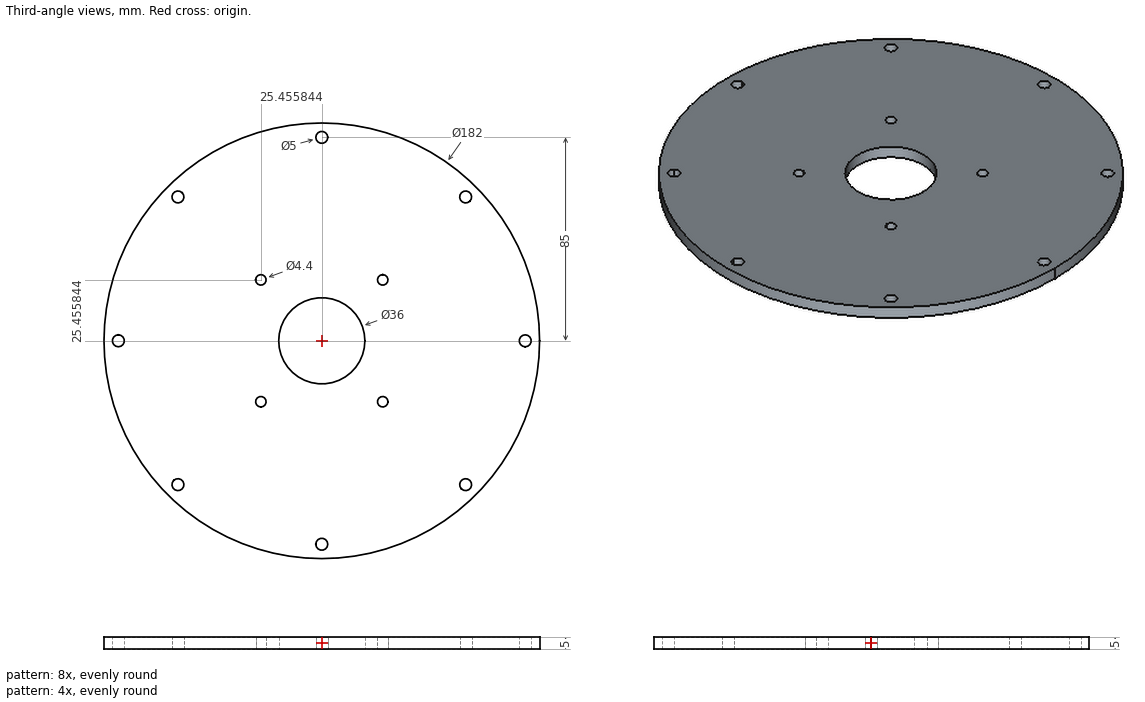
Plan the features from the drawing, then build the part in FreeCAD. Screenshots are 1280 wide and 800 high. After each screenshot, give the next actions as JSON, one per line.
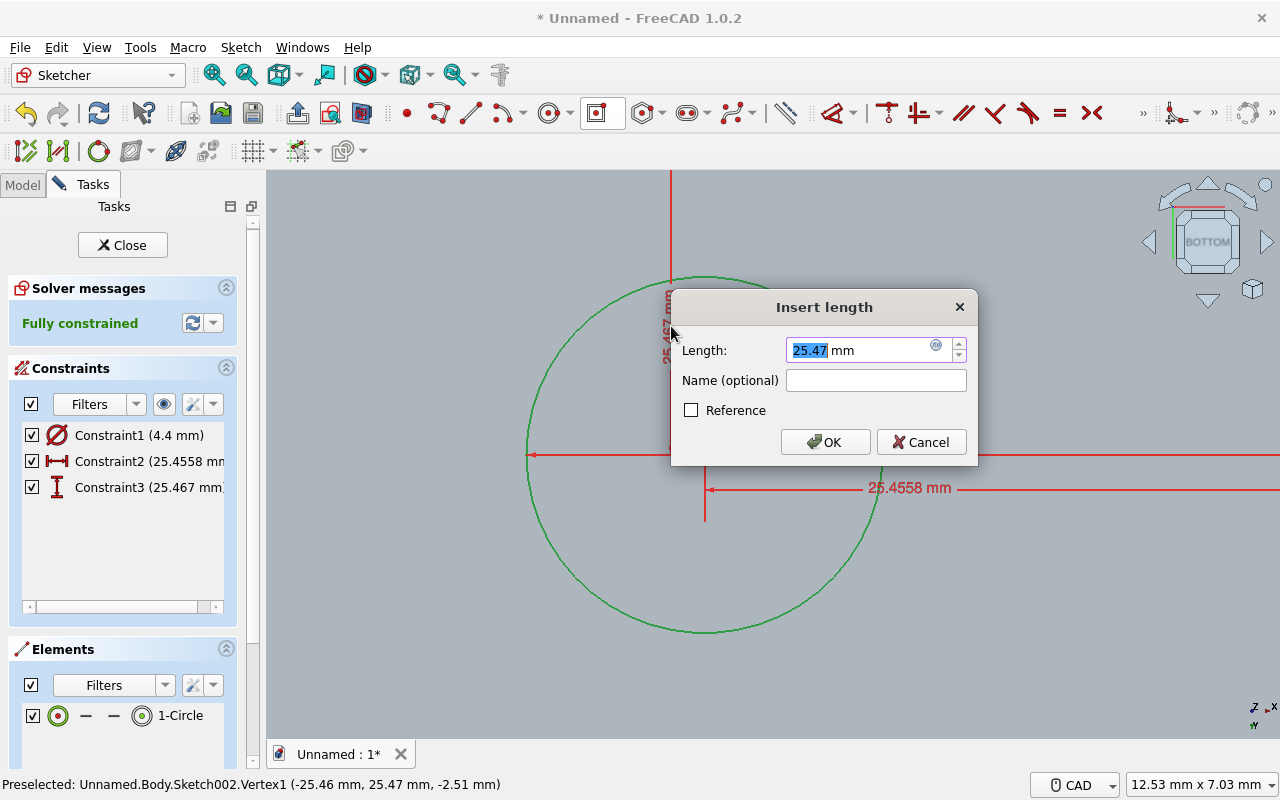
{"action": "type", "text": "25.455844"}
{"action": "key", "text": "Return"}
{"action": "key", "text": "Escape"}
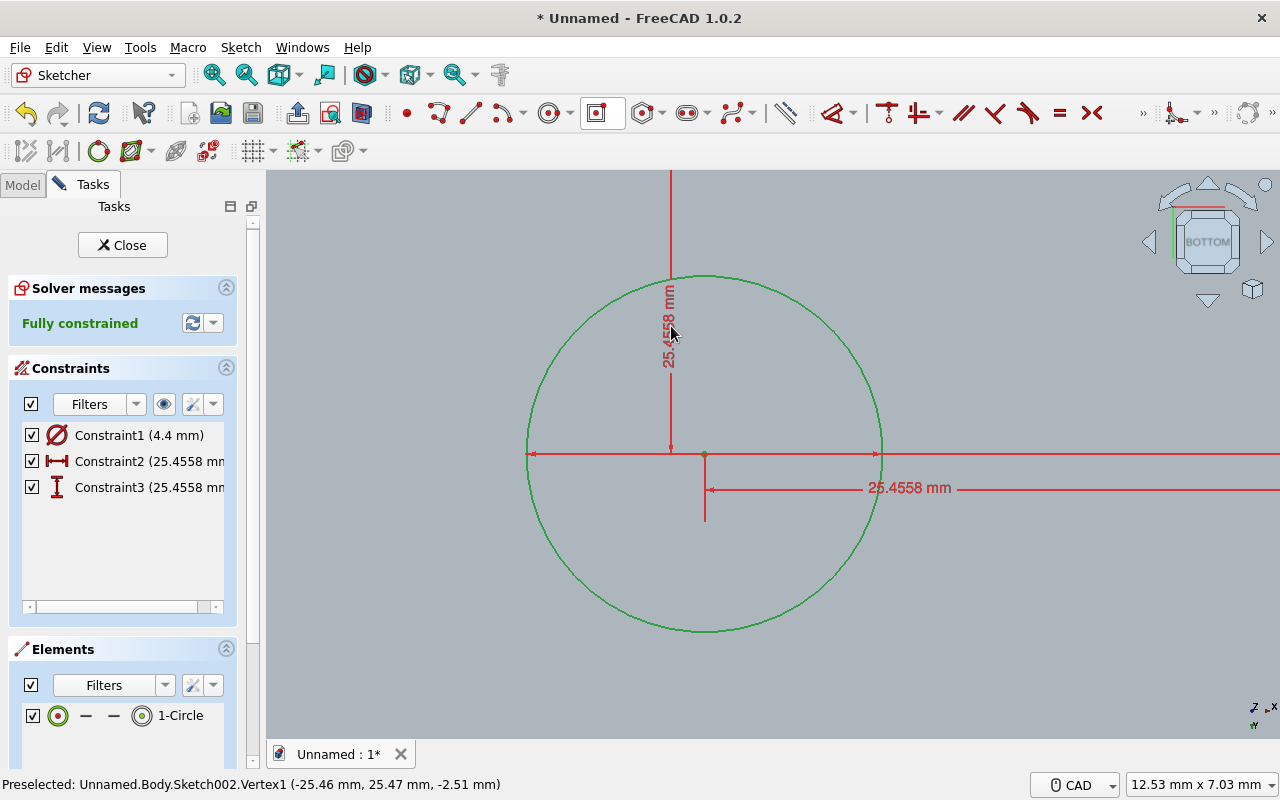
{"action": "left_click", "coordinate": [123, 245]}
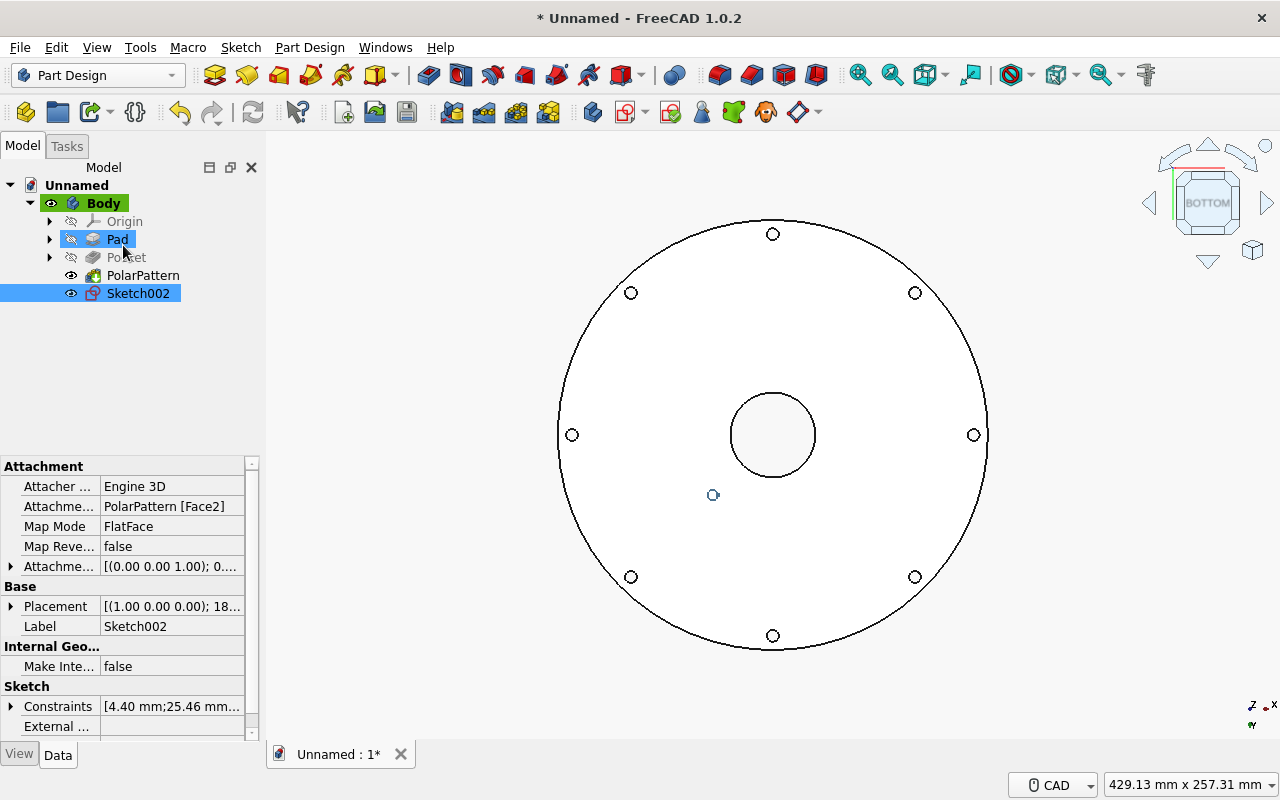
{"action": "left_click", "coordinate": [430, 76]}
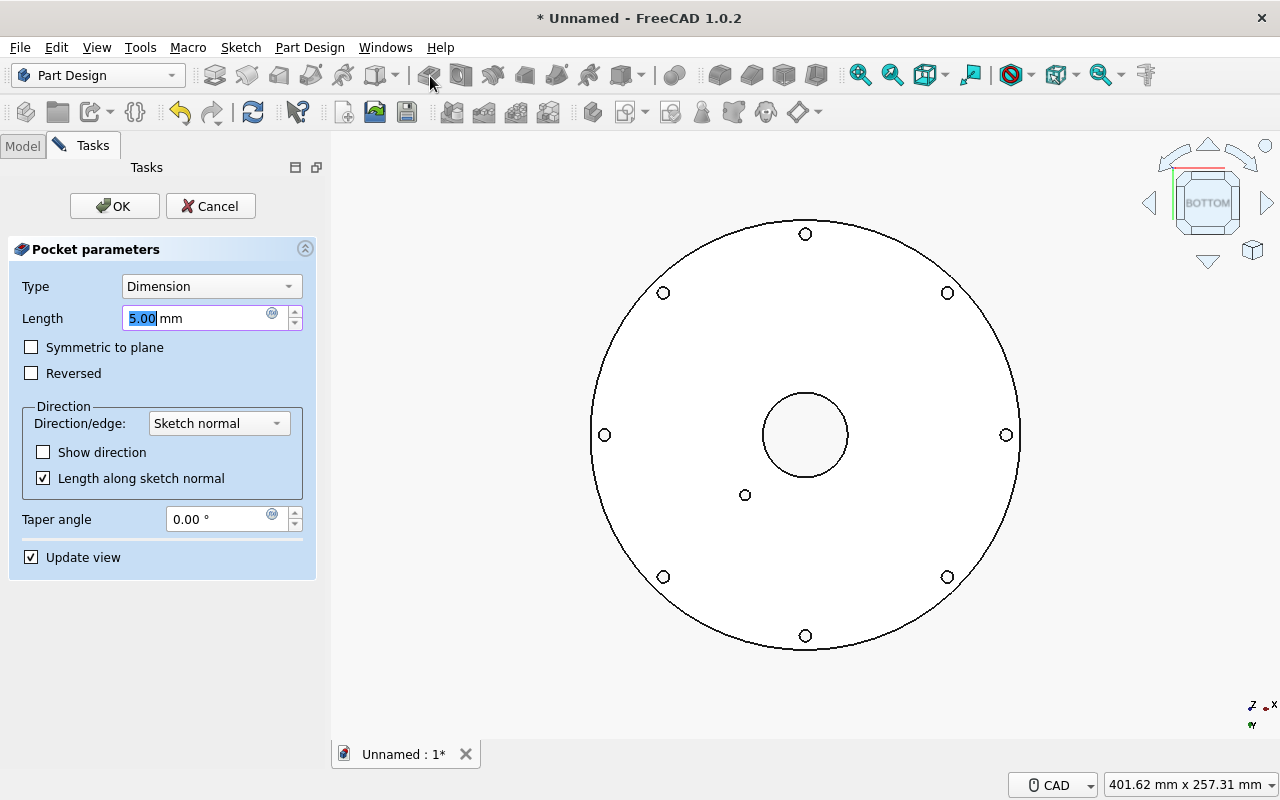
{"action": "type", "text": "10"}
{"action": "key", "text": "Tab"}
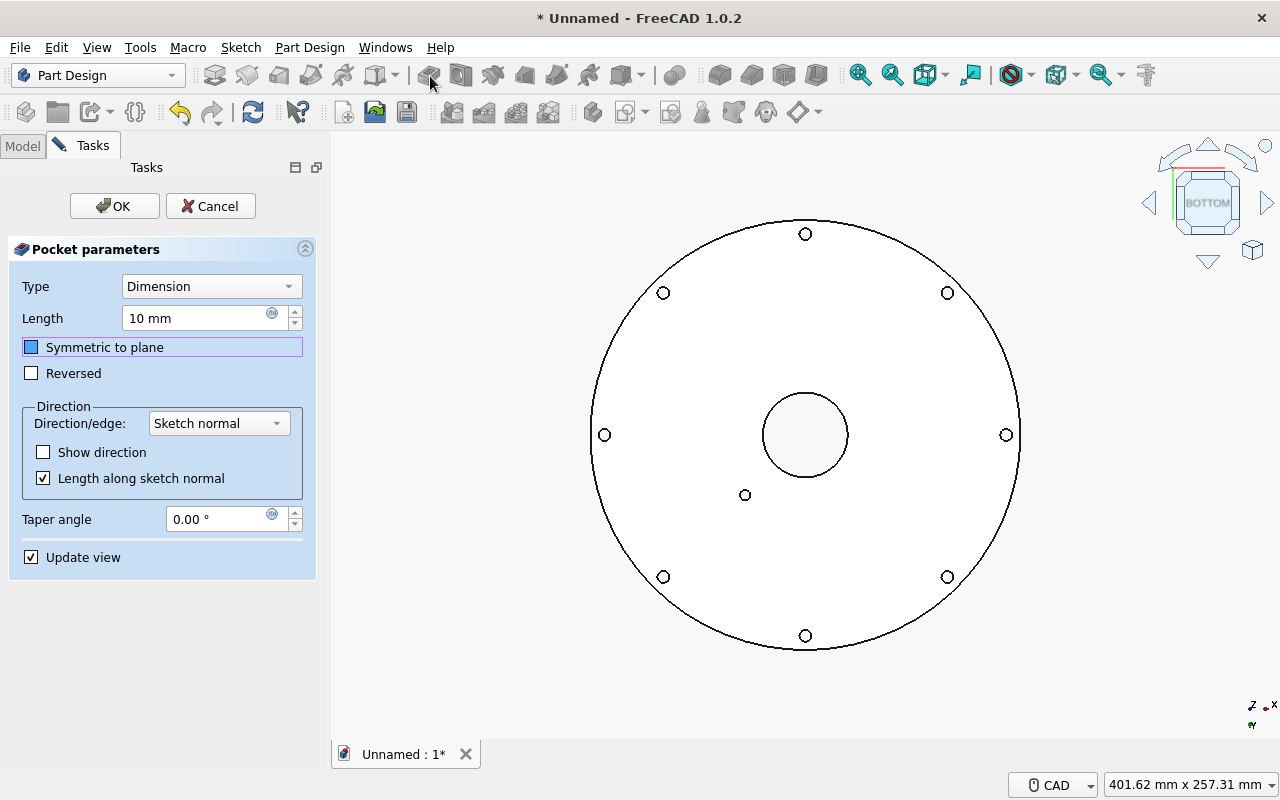
{"action": "left_click", "coordinate": [115, 206]}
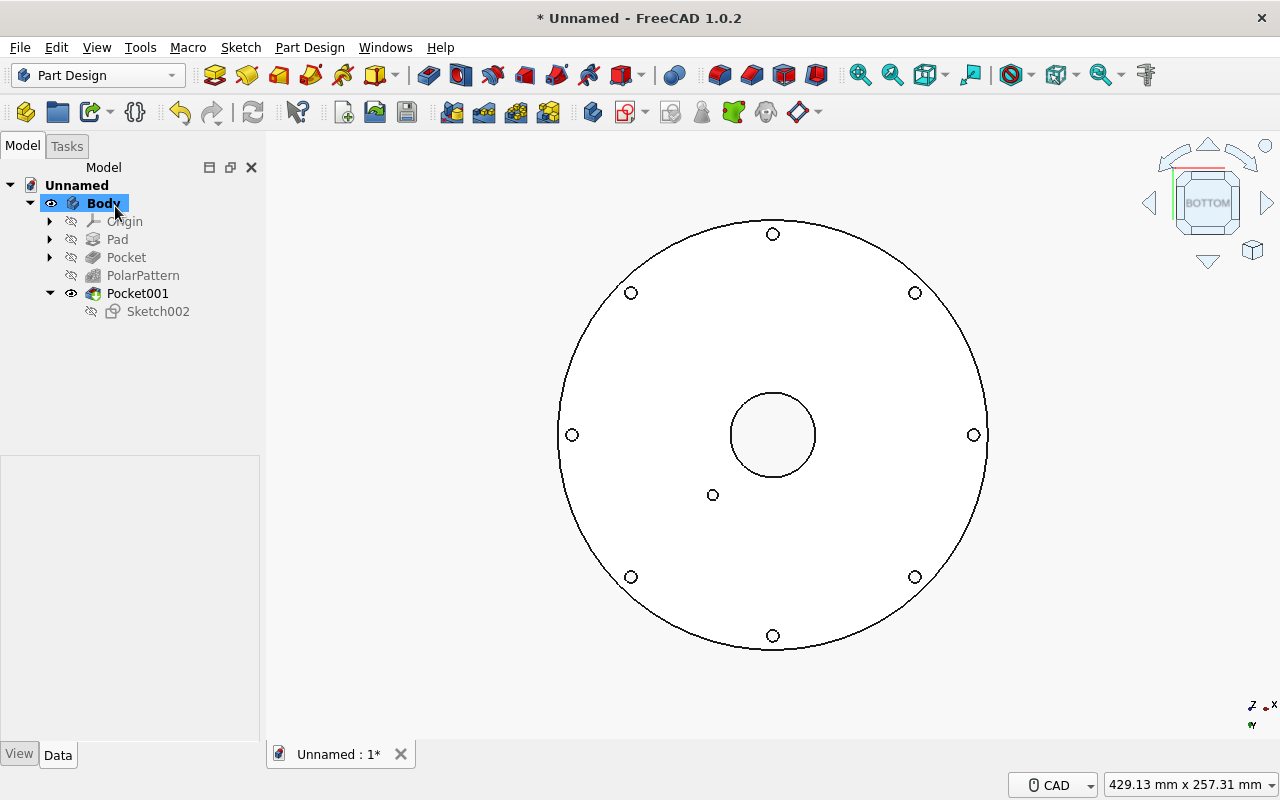
{"action": "left_click", "coordinate": [116, 293]}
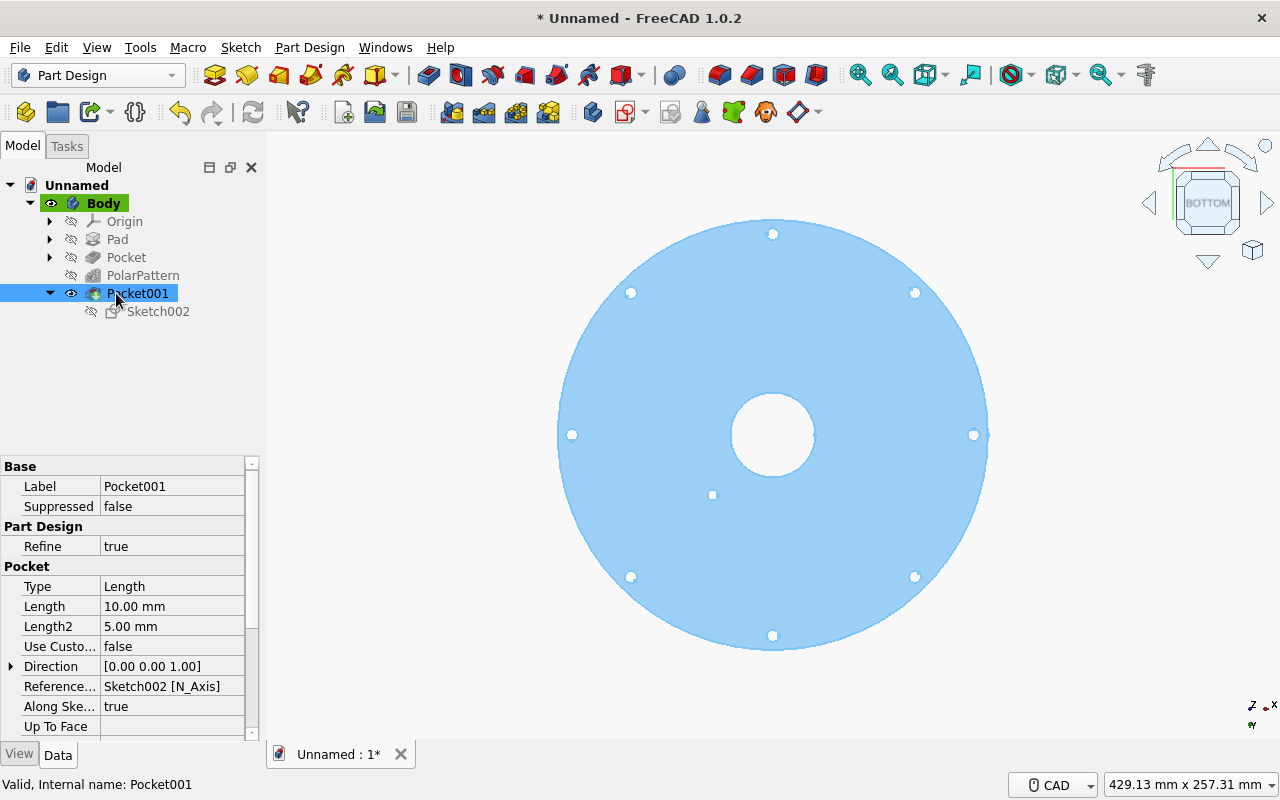
{"action": "left_click", "coordinate": [516, 112]}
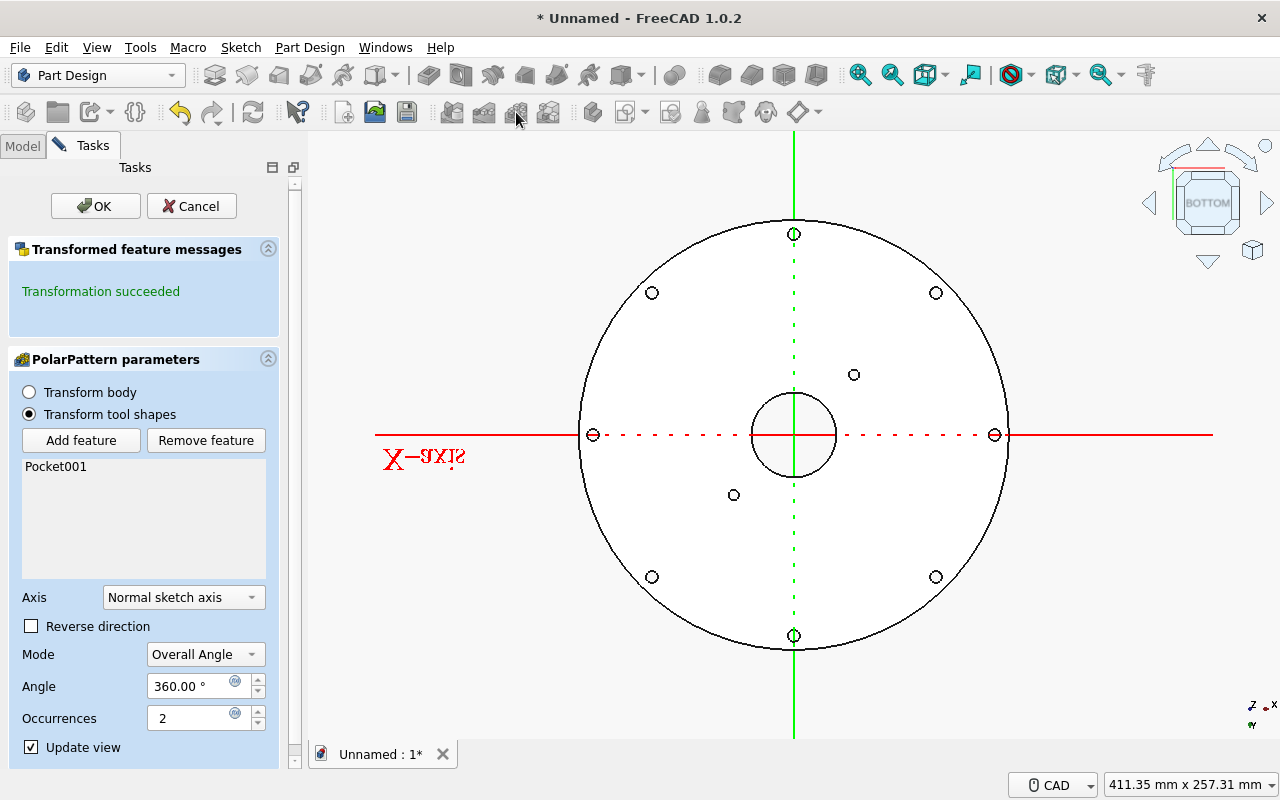
{"action": "left_click", "coordinate": [184, 598]}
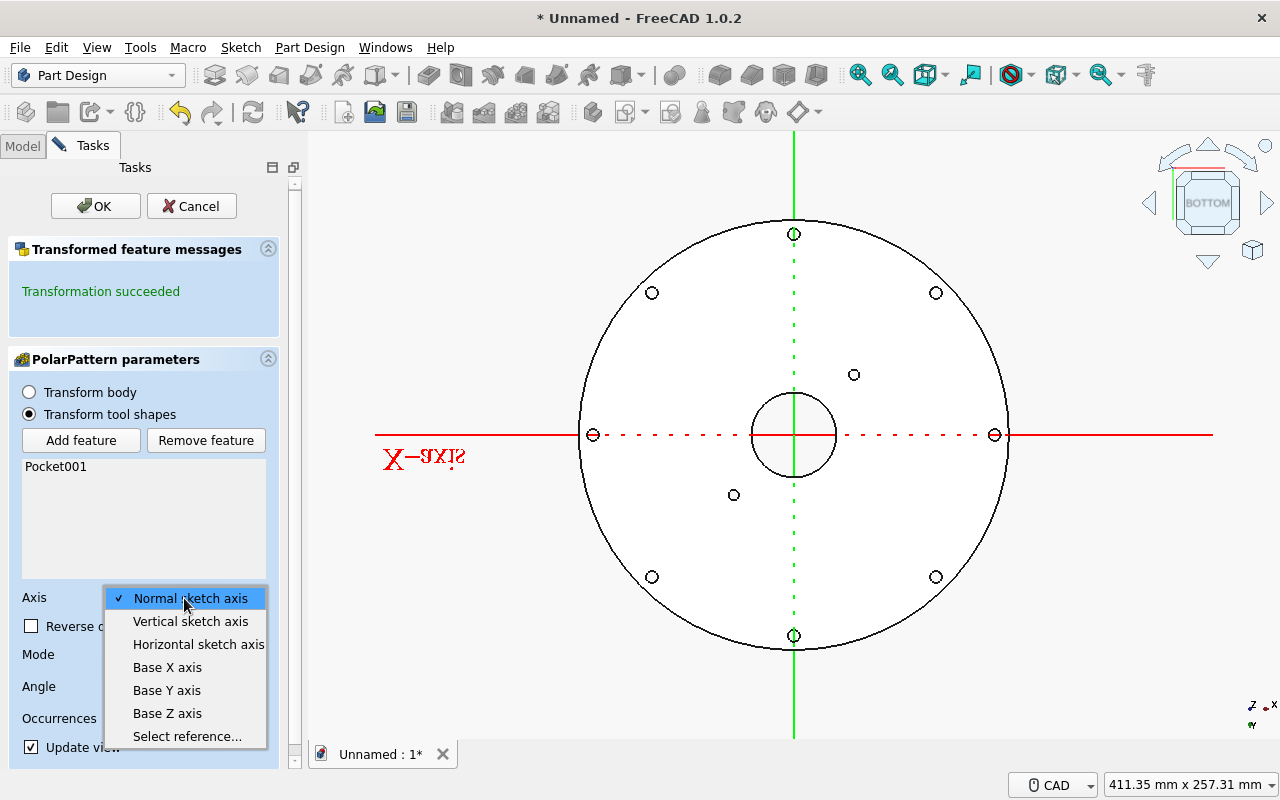
{"action": "left_click", "coordinate": [184, 714]}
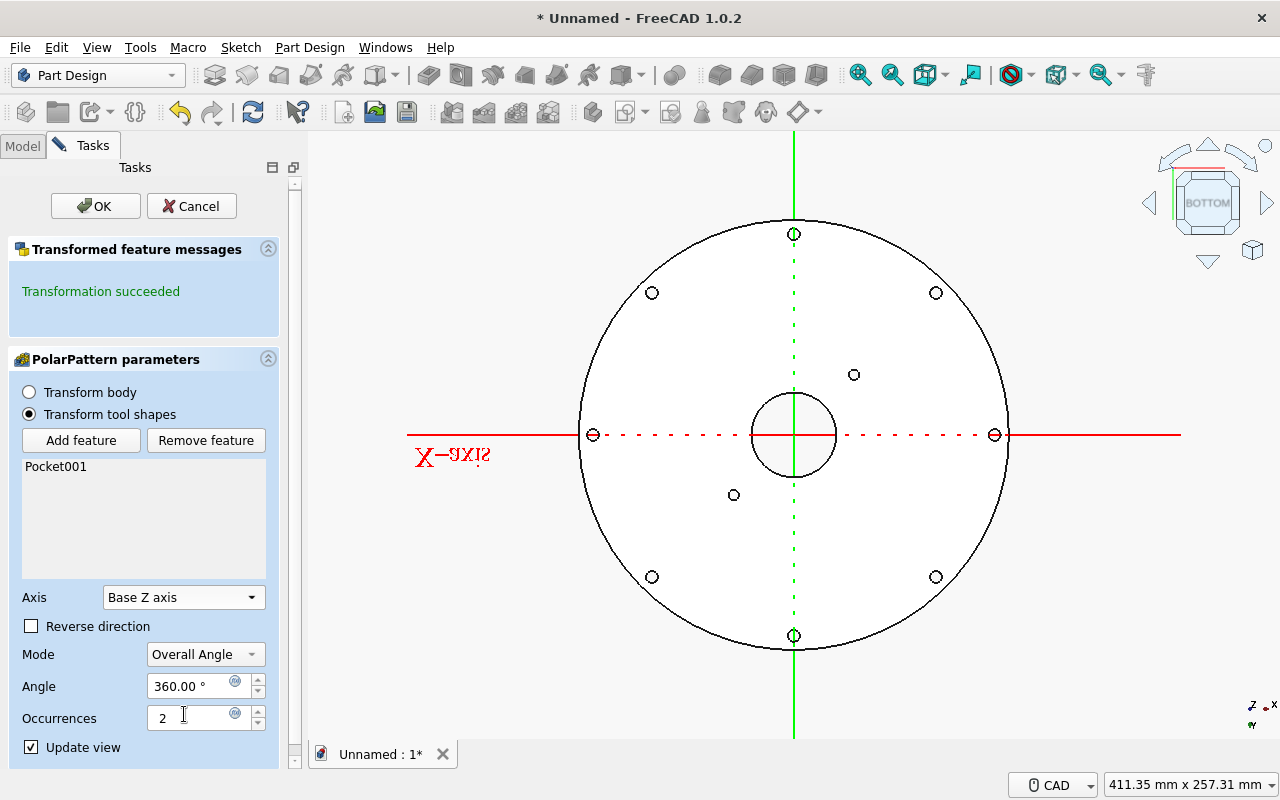
{"action": "triple_click", "coordinate": [198, 718]}